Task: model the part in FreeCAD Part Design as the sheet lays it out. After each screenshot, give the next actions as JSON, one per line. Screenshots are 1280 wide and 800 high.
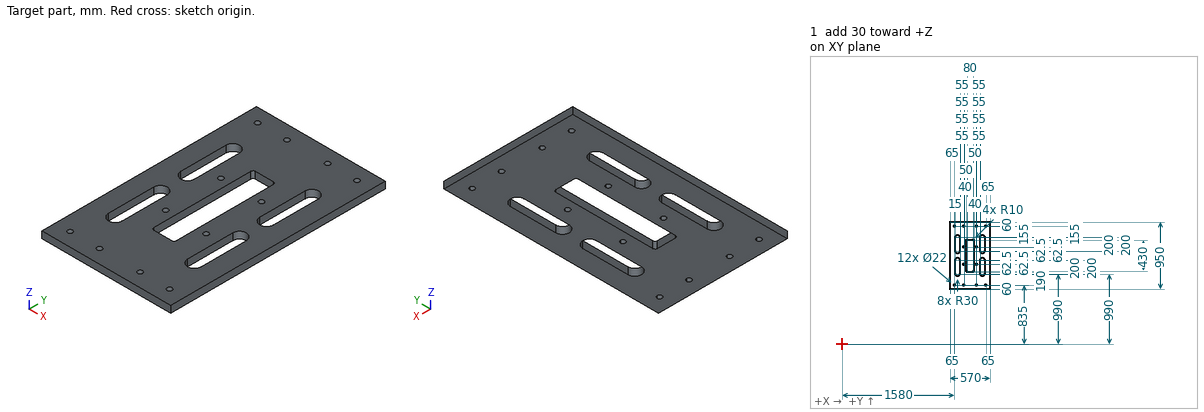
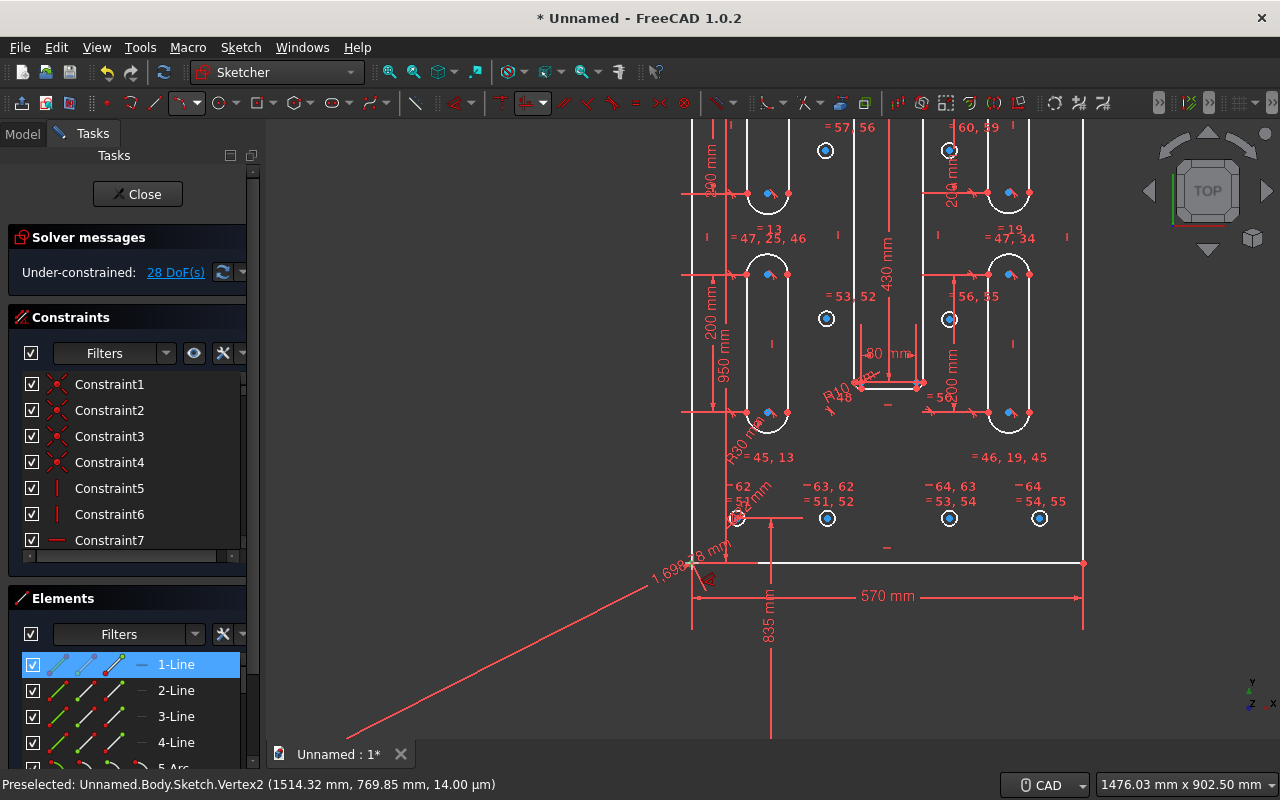
{"action": "left_click", "coordinate": [737, 518]}
{"action": "left_click", "coordinate": [699, 597]}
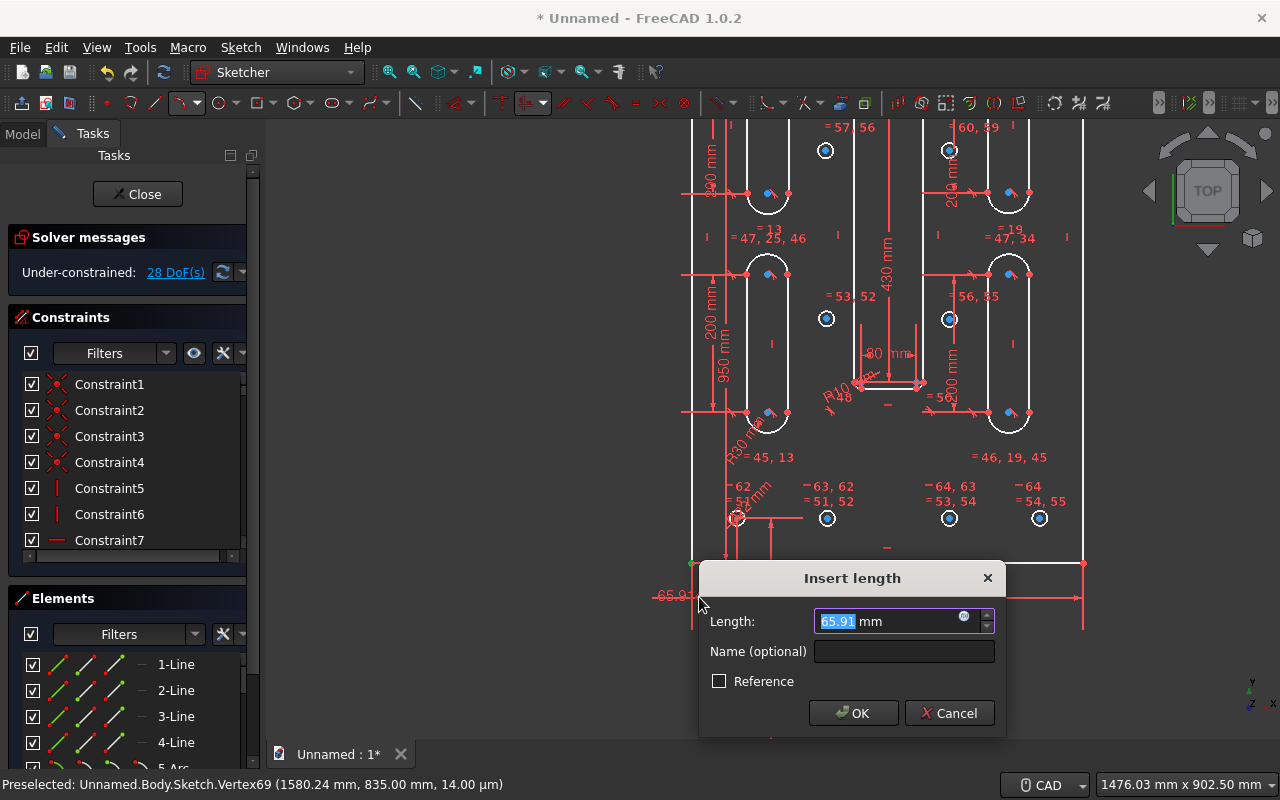
{"action": "type", "text": "65"}
{"action": "key", "text": "Return"}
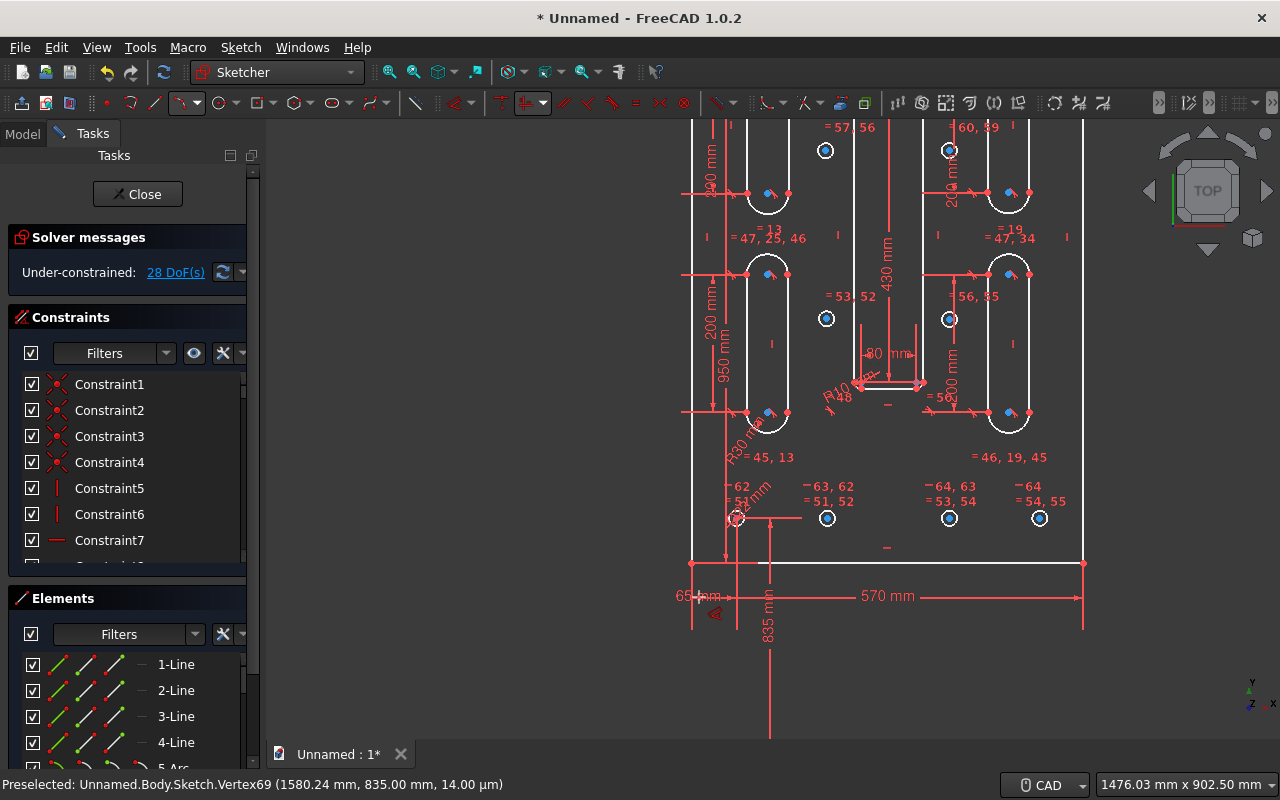
{"action": "scroll", "coordinate": [747, 412], "scroll_direction": "up", "scroll_amount": 7}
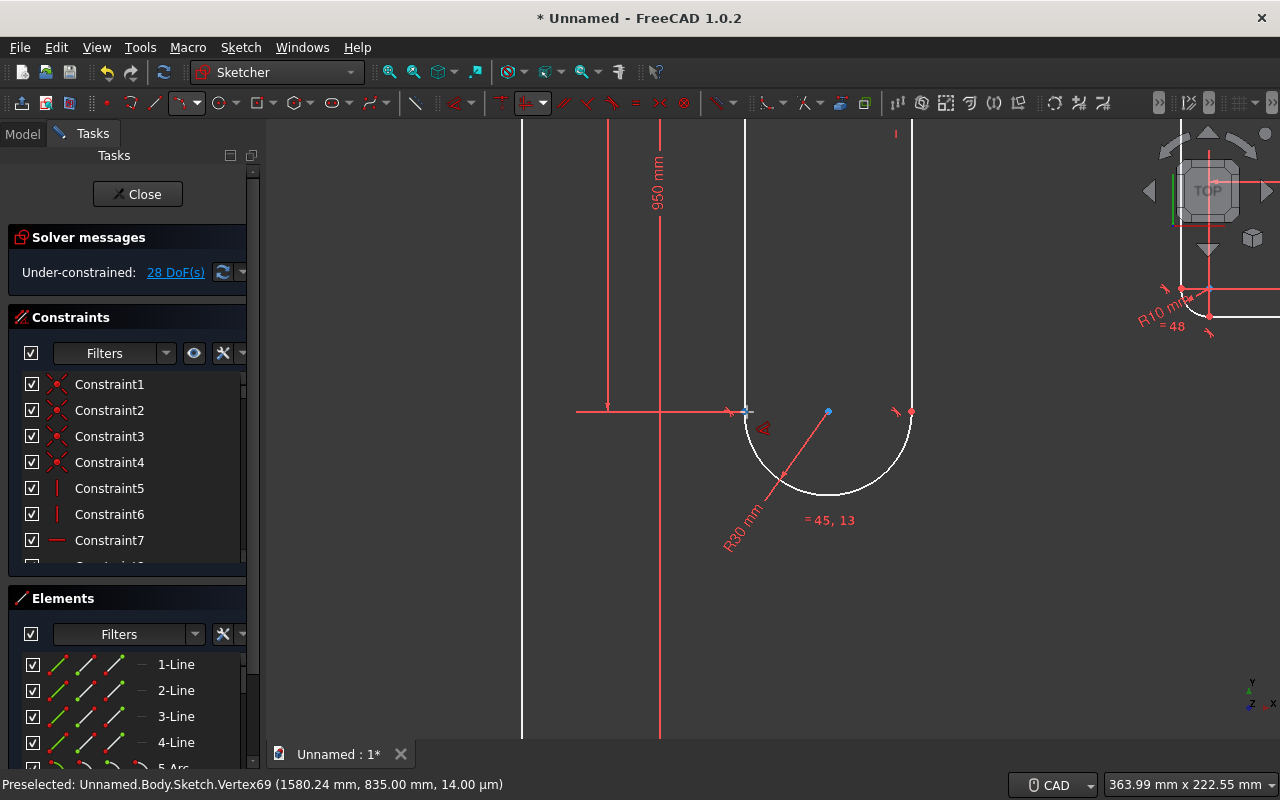
{"action": "left_click", "coordinate": [745, 412]}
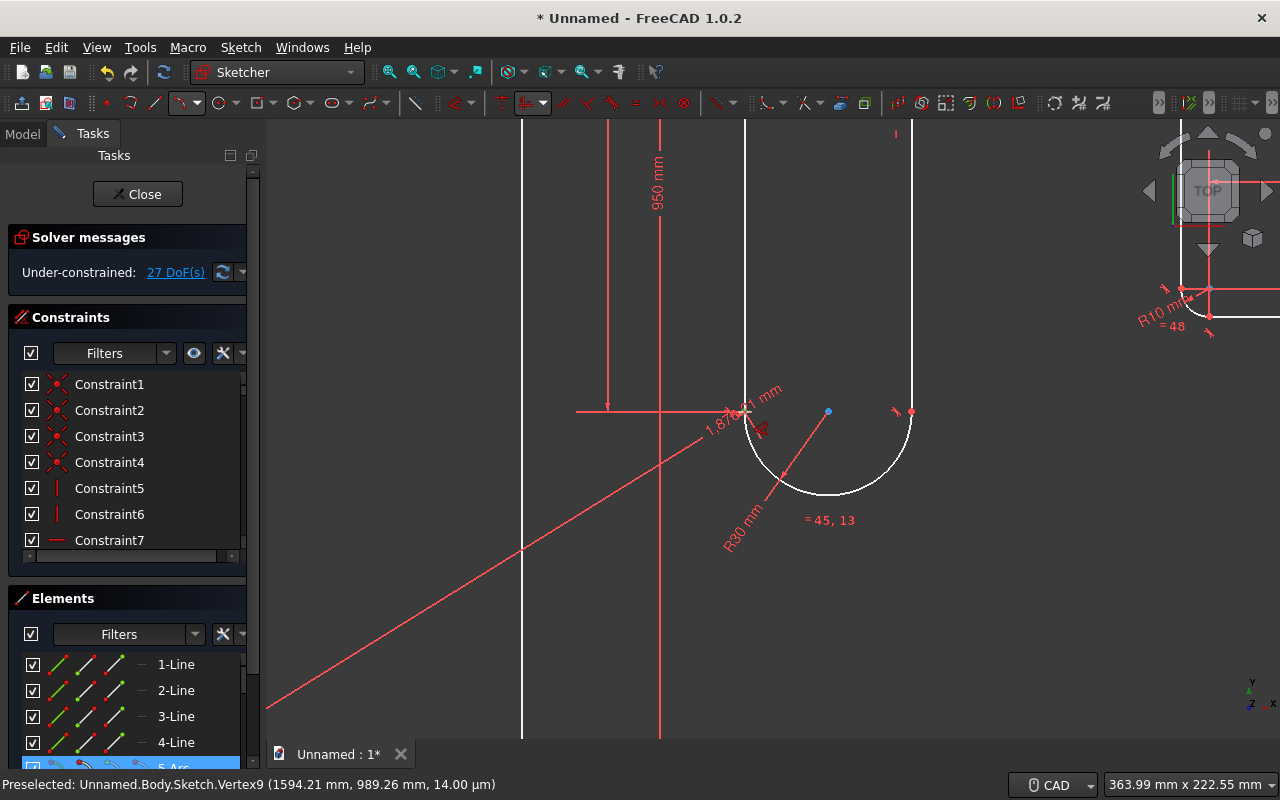
{"action": "scroll", "coordinate": [854, 395], "scroll_direction": "down", "scroll_amount": 12}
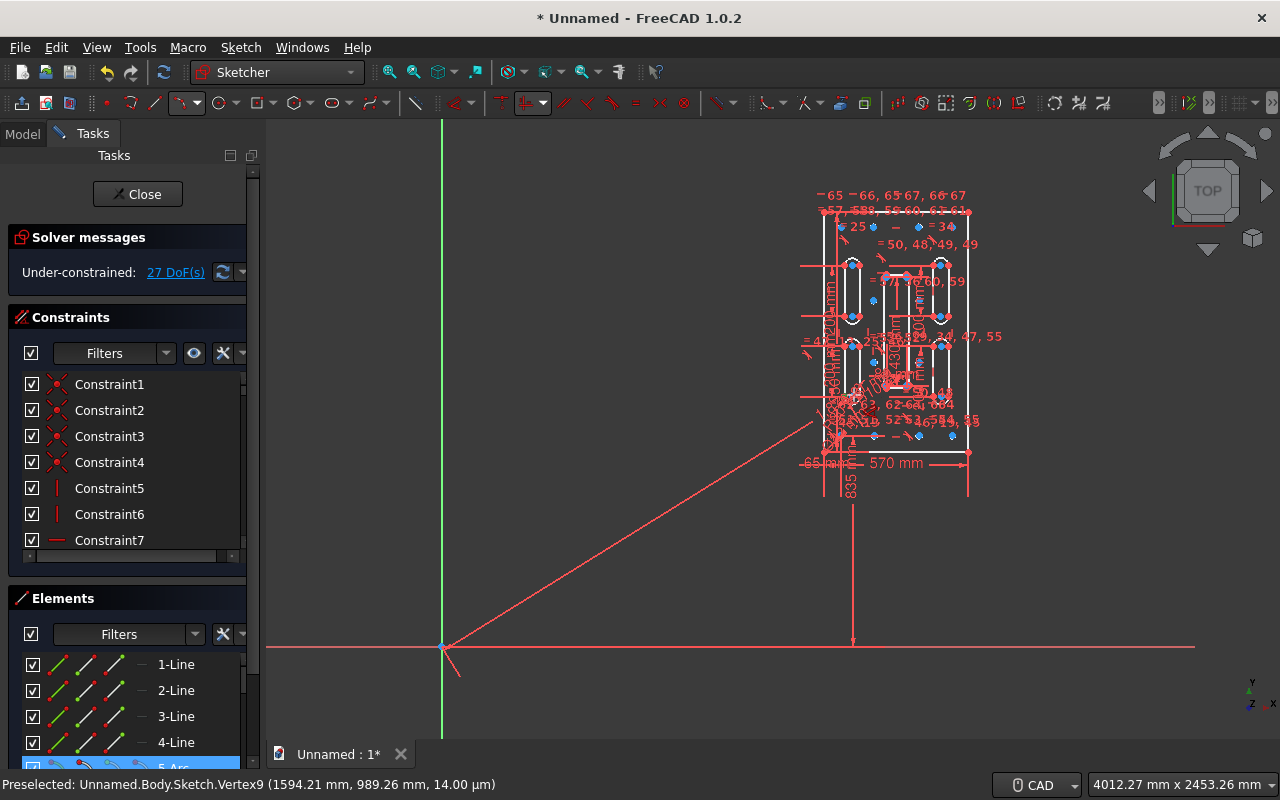
{"action": "scroll", "coordinate": [841, 436], "scroll_direction": "up", "scroll_amount": 12}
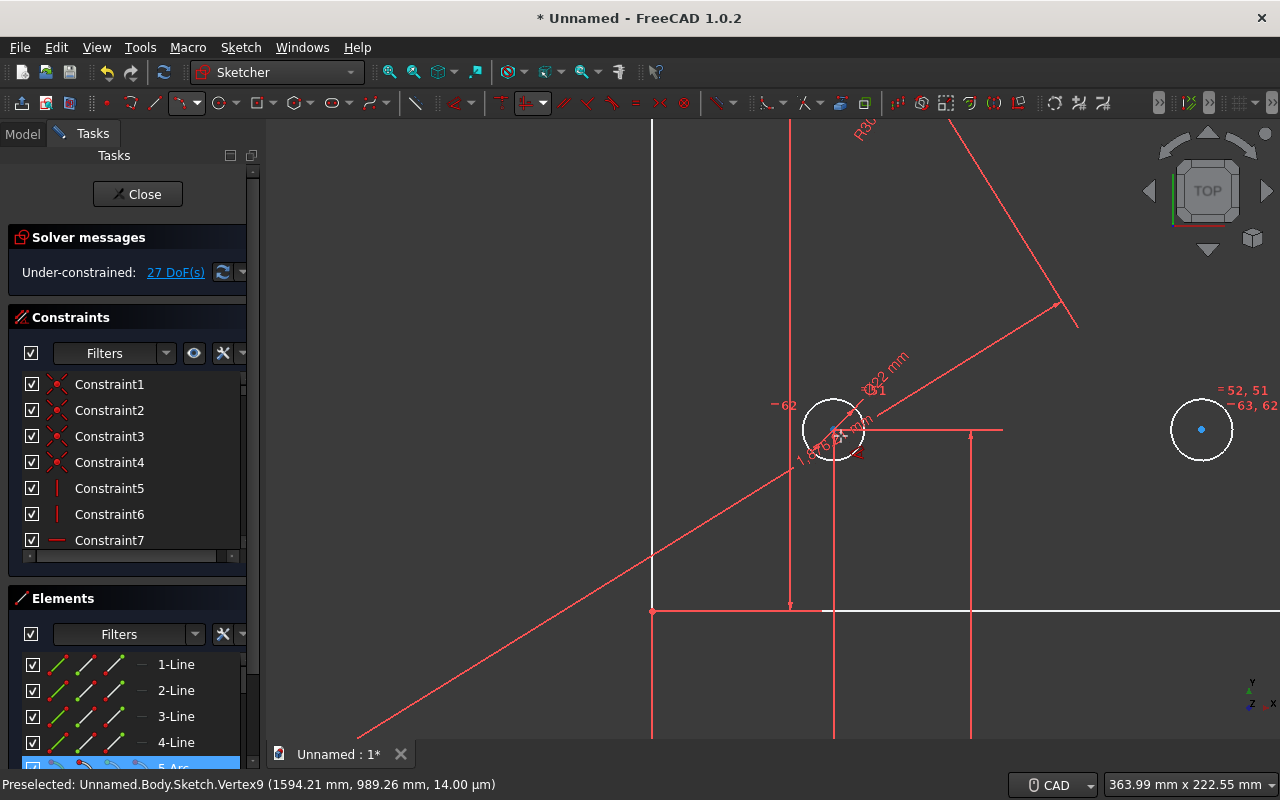
{"action": "left_click", "coordinate": [834, 430]}
{"action": "left_click", "coordinate": [864, 464]}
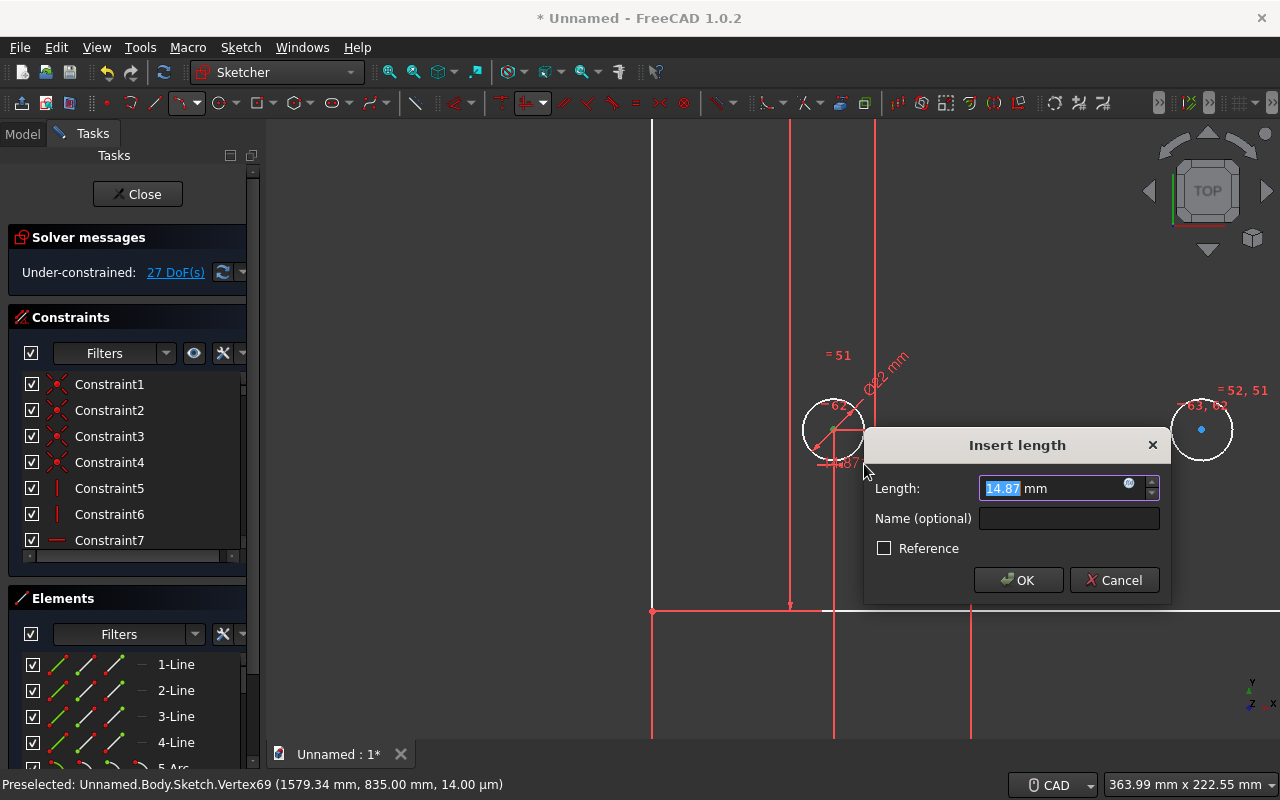
{"action": "type", "text": "15"}
{"action": "key", "text": "Return"}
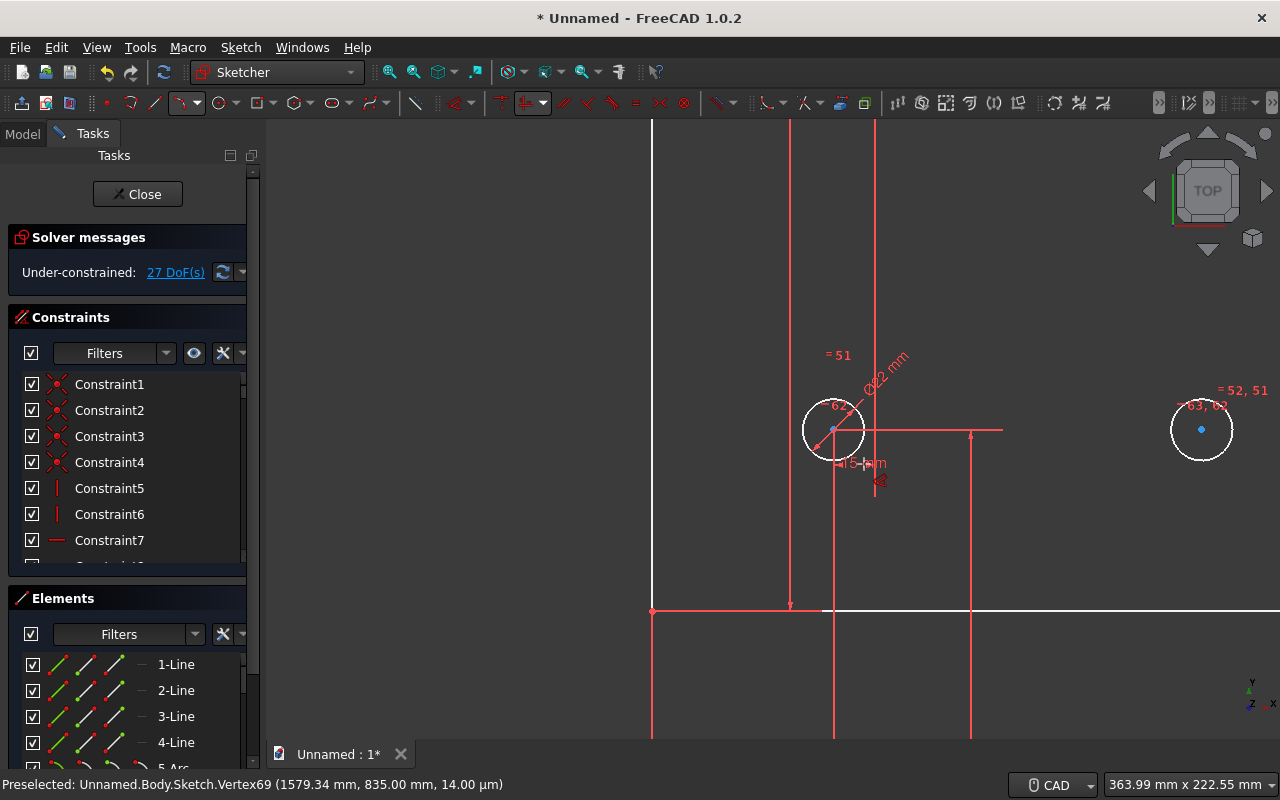
{"action": "scroll", "coordinate": [841, 437], "scroll_direction": "down", "scroll_amount": 12}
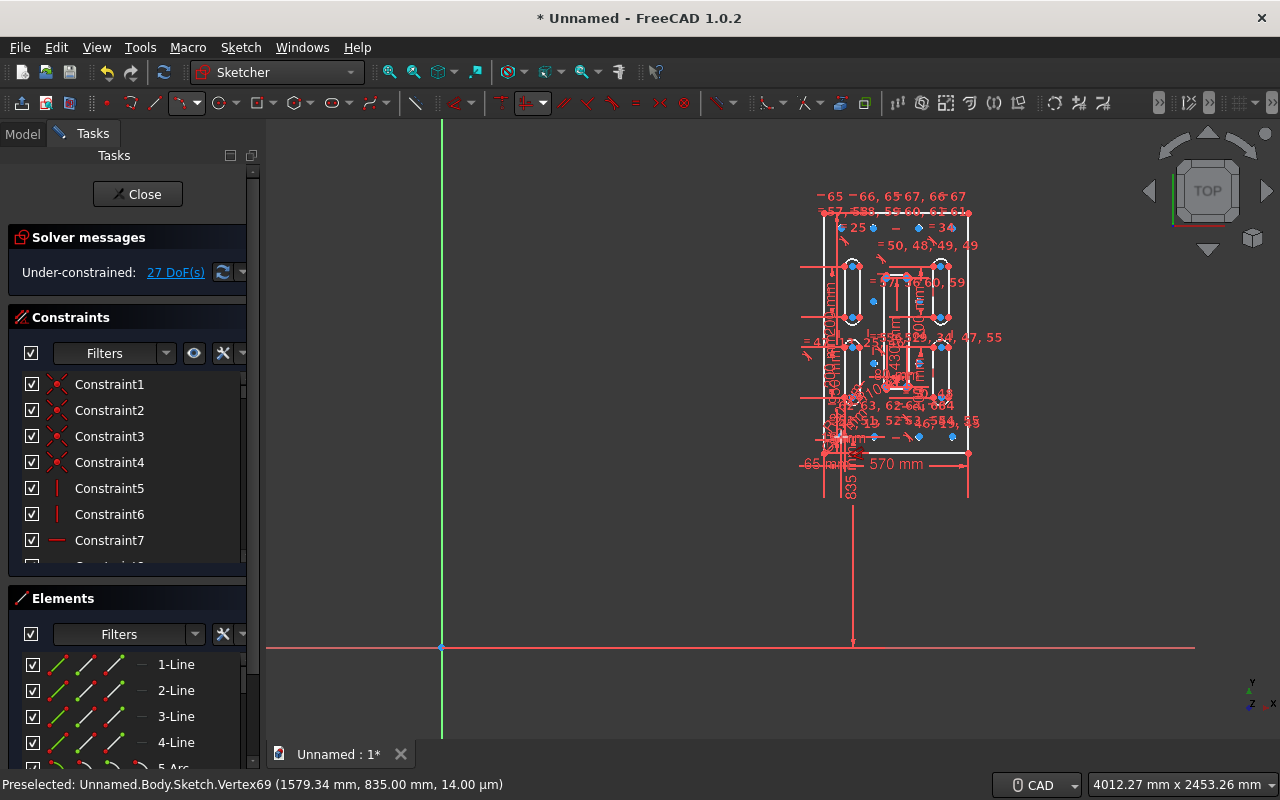
{"action": "scroll", "coordinate": [824, 453], "scroll_direction": "up", "scroll_amount": 5}